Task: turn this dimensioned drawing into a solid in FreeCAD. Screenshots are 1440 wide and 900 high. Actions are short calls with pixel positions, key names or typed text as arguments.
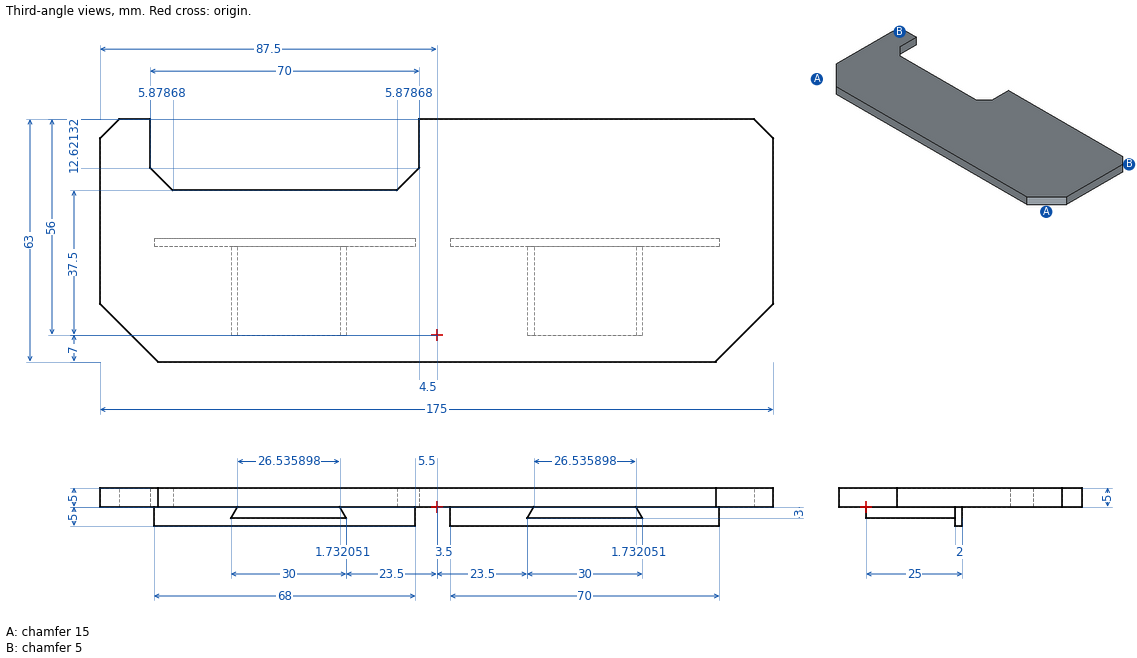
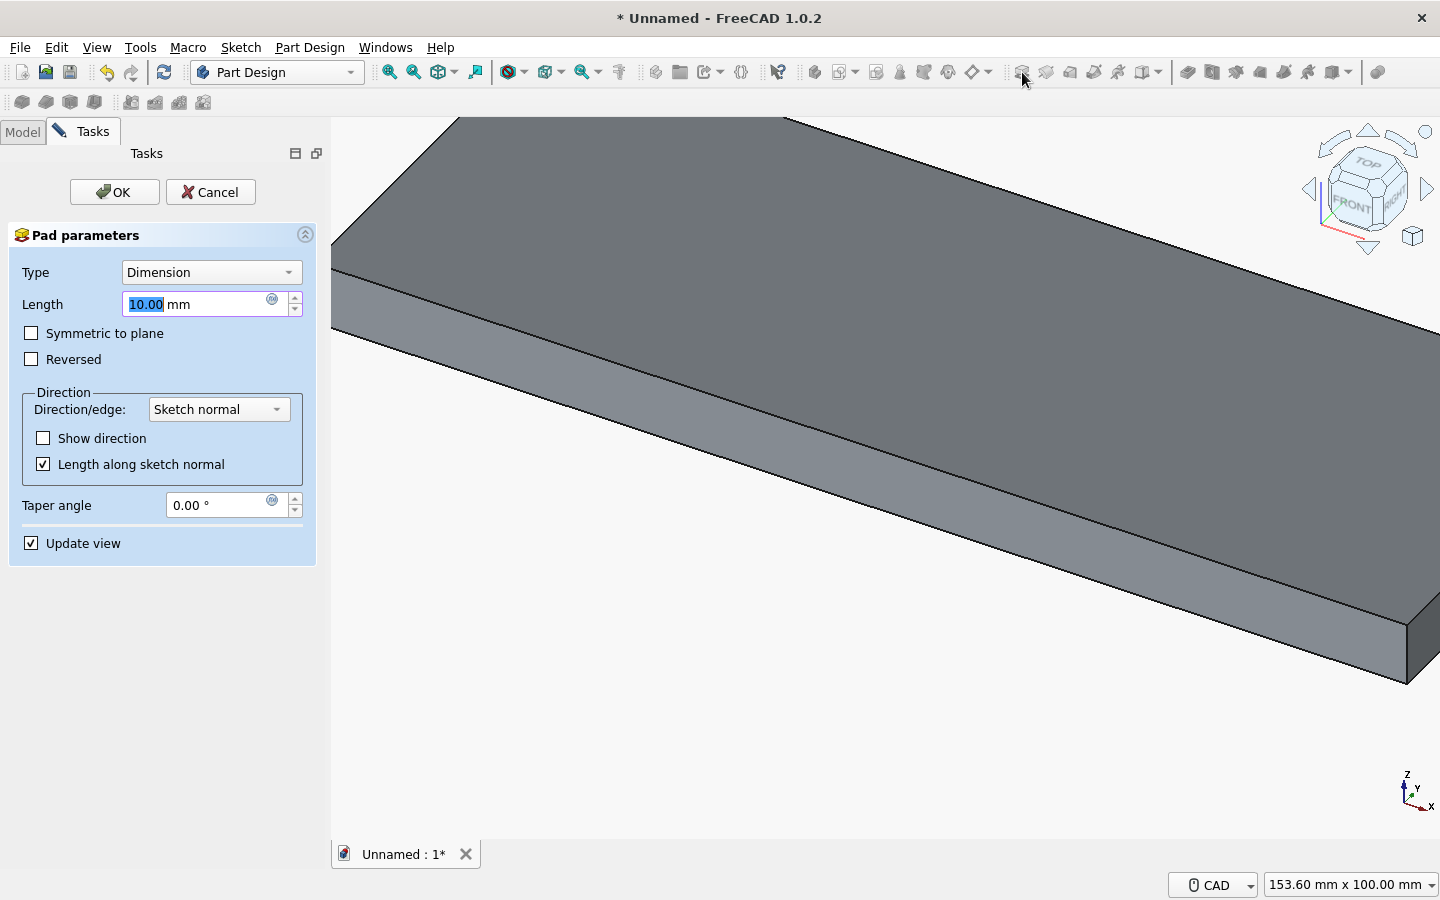
text(5)
key(Tab)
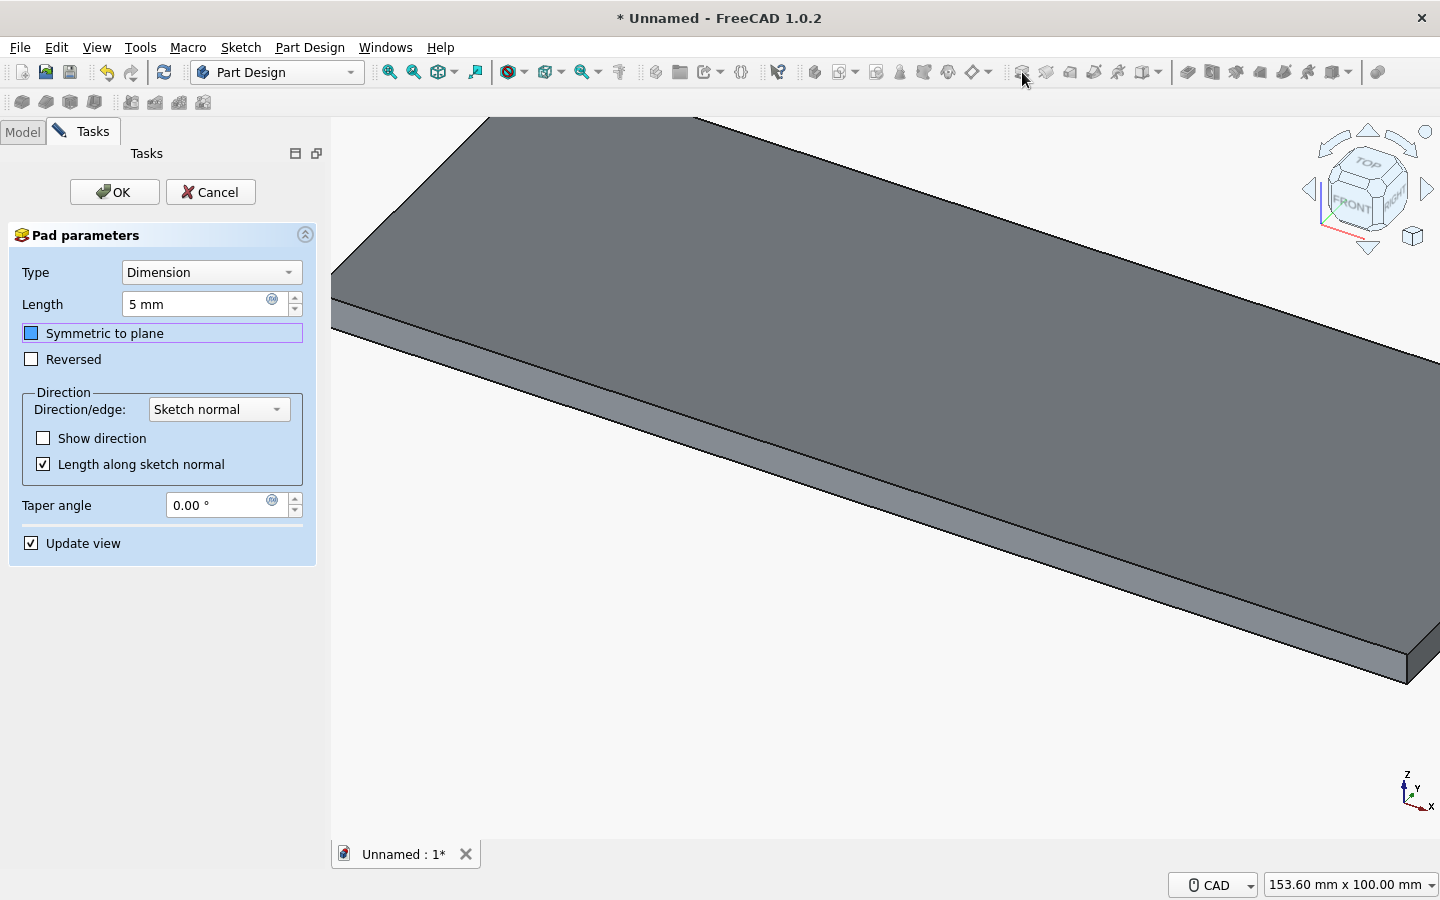
click(115, 192)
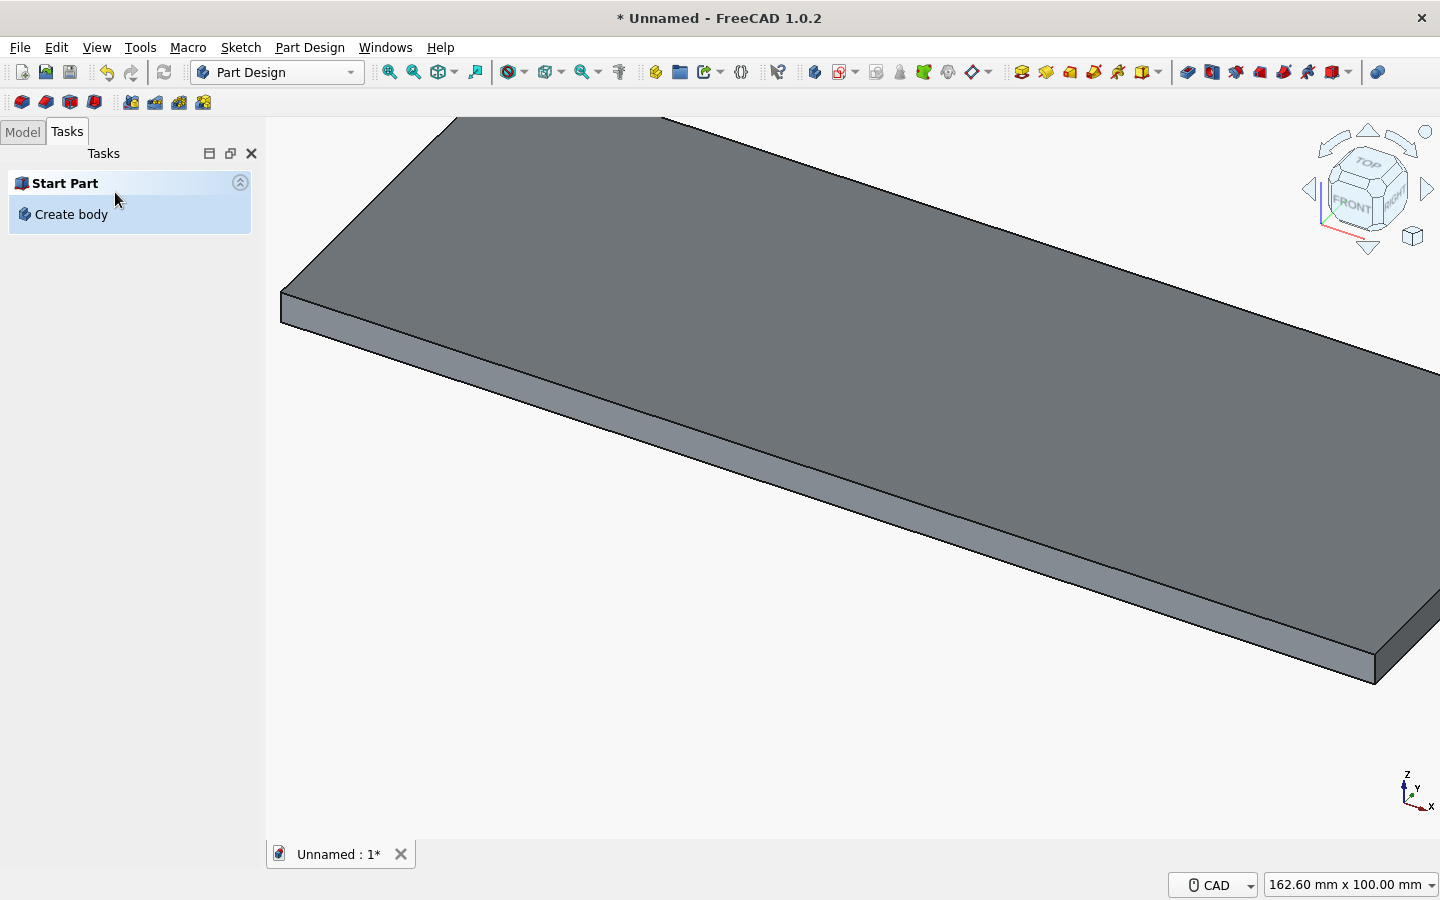
click(390, 72)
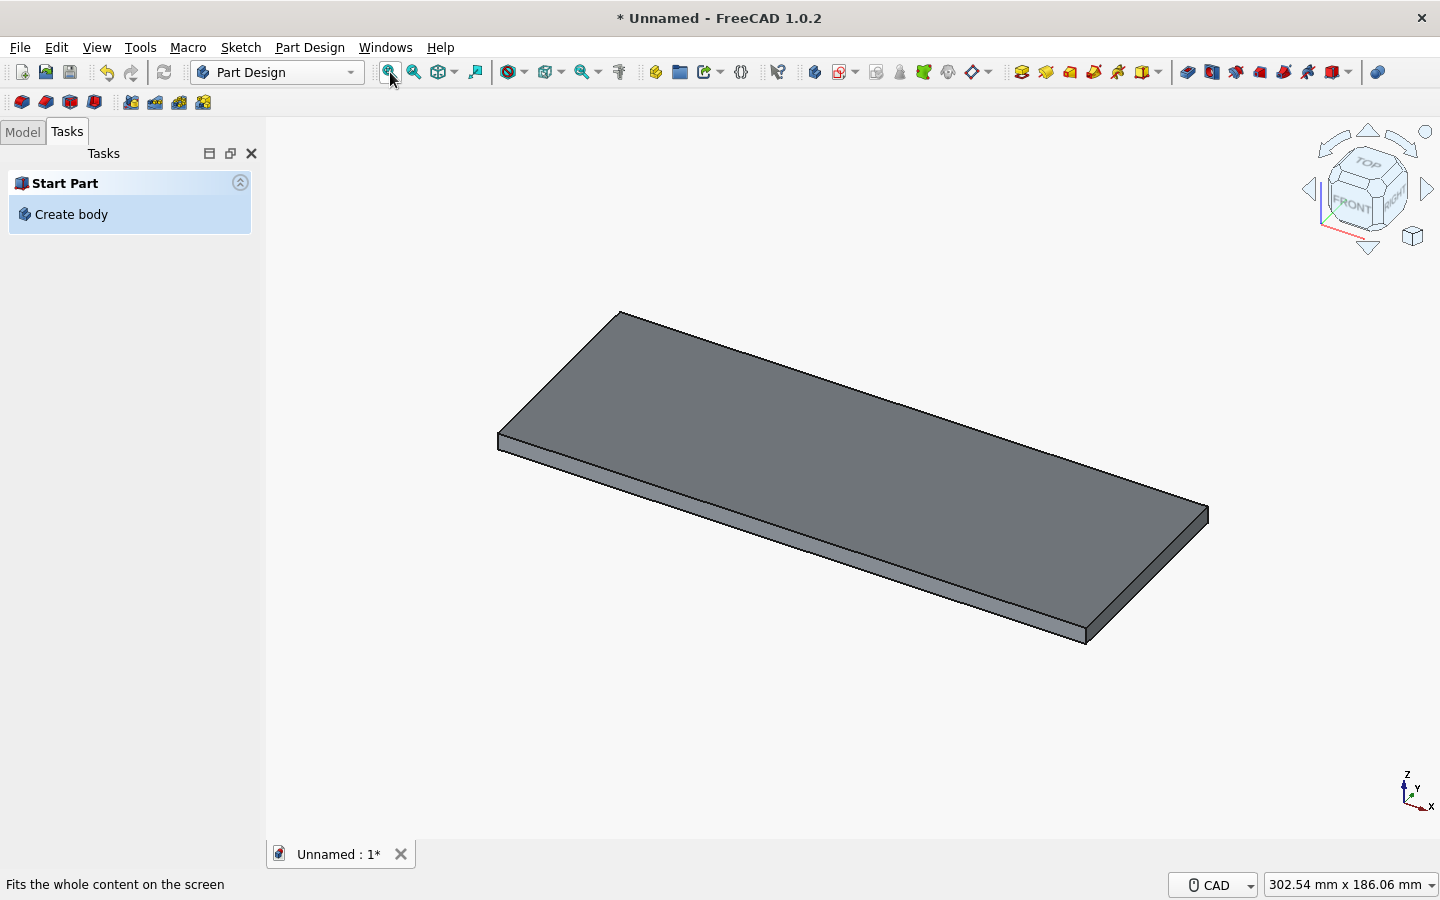
click(1021, 525)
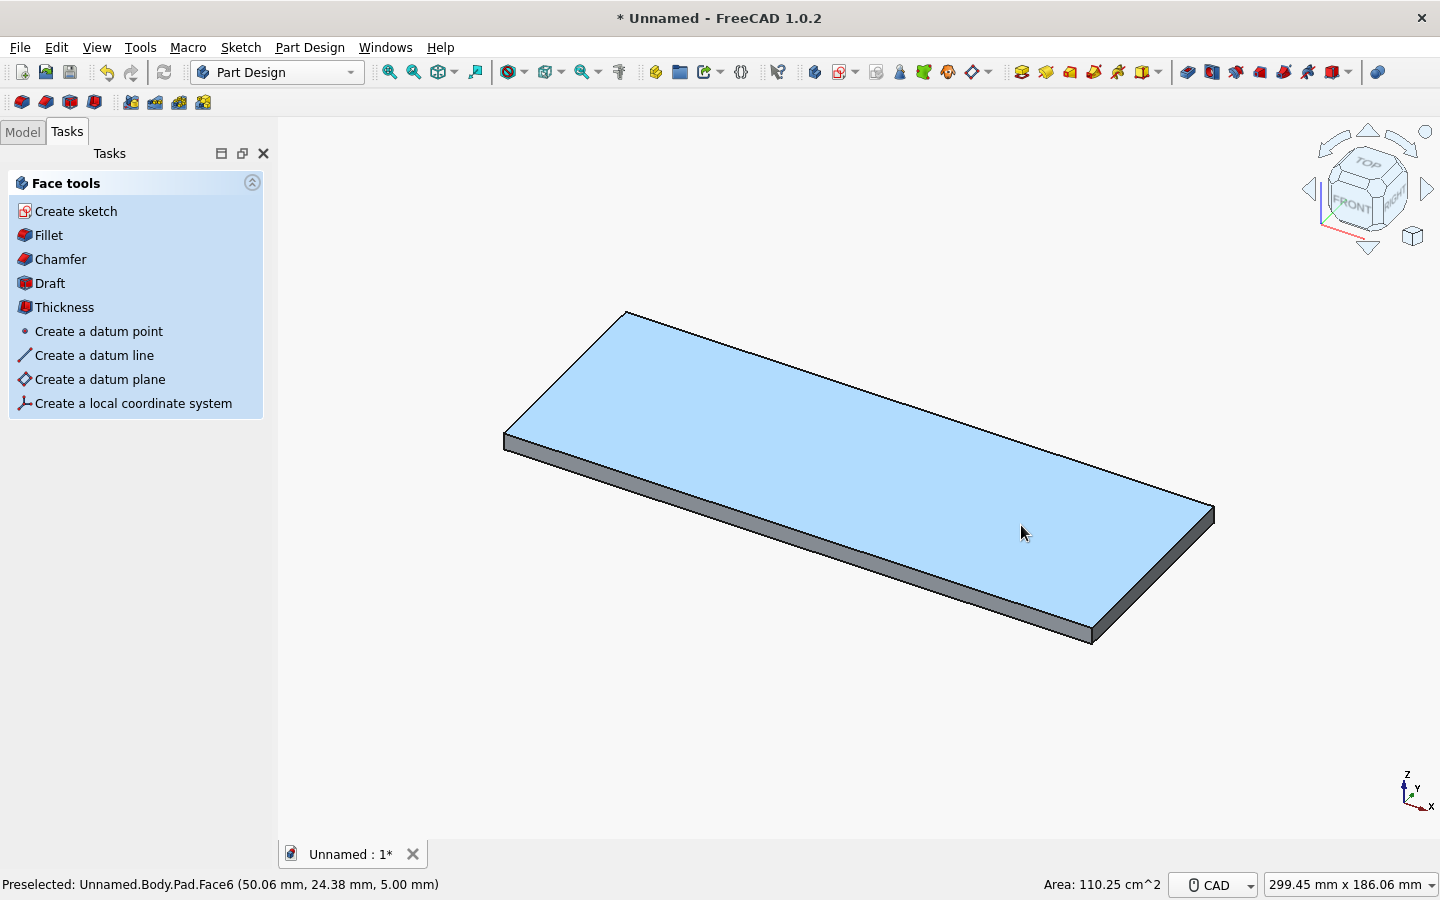
click(840, 72)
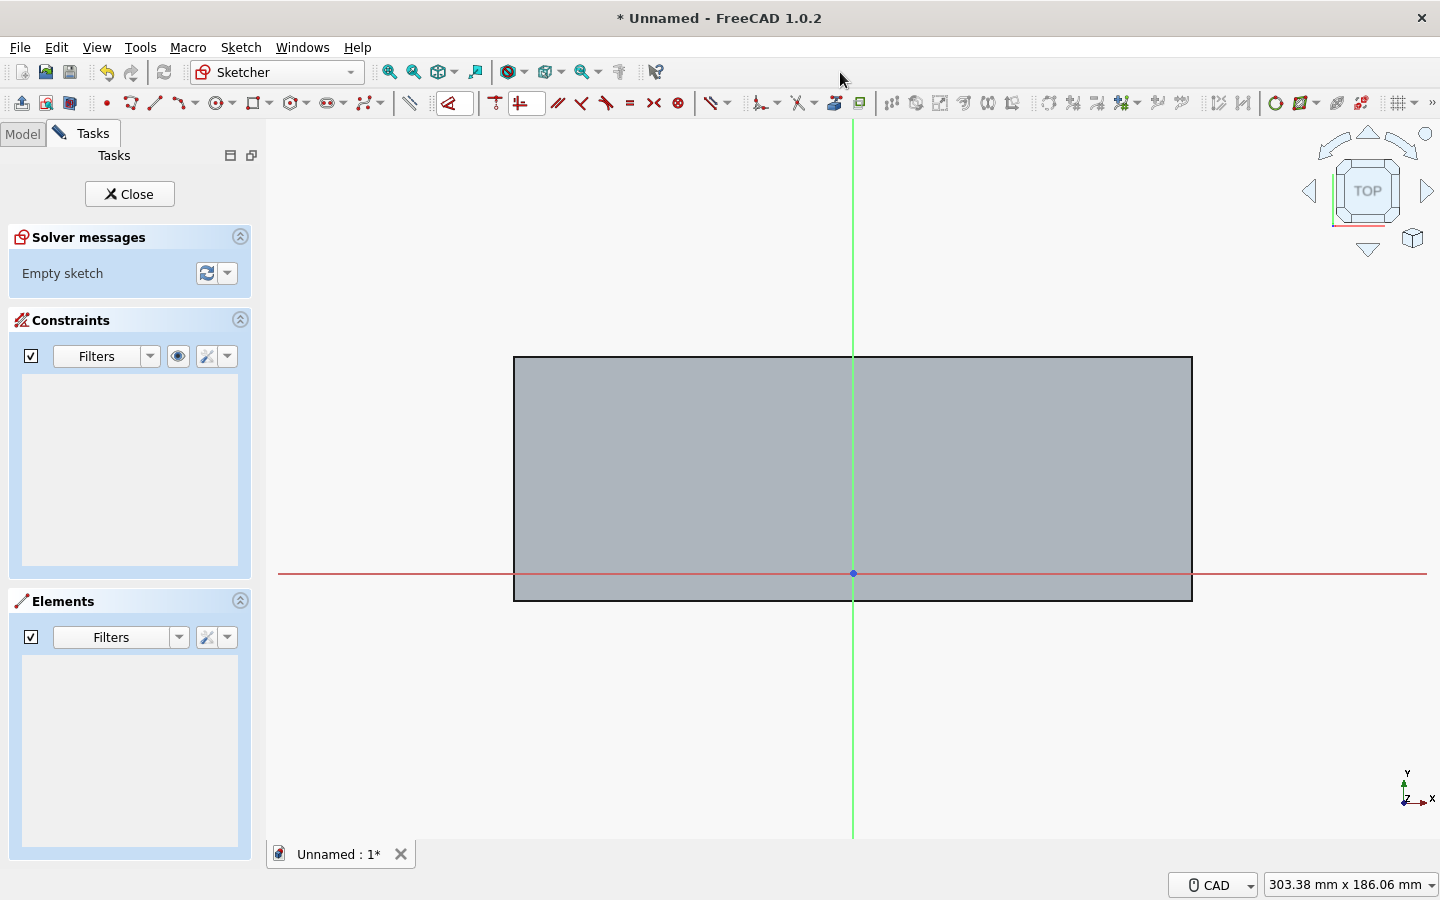
scroll(647, 454, up, 4)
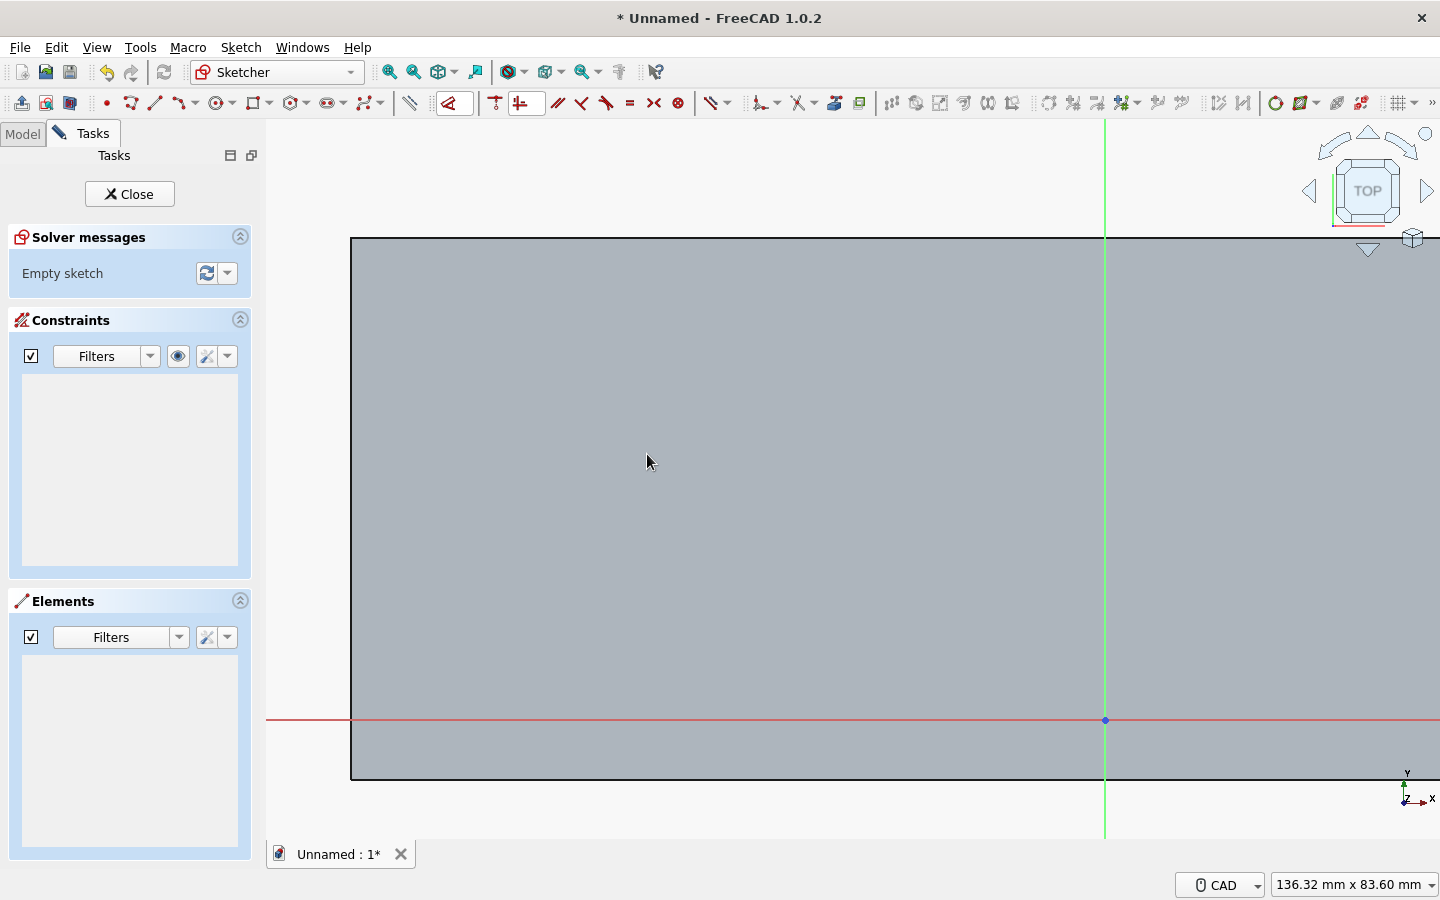
key(g)
key(m)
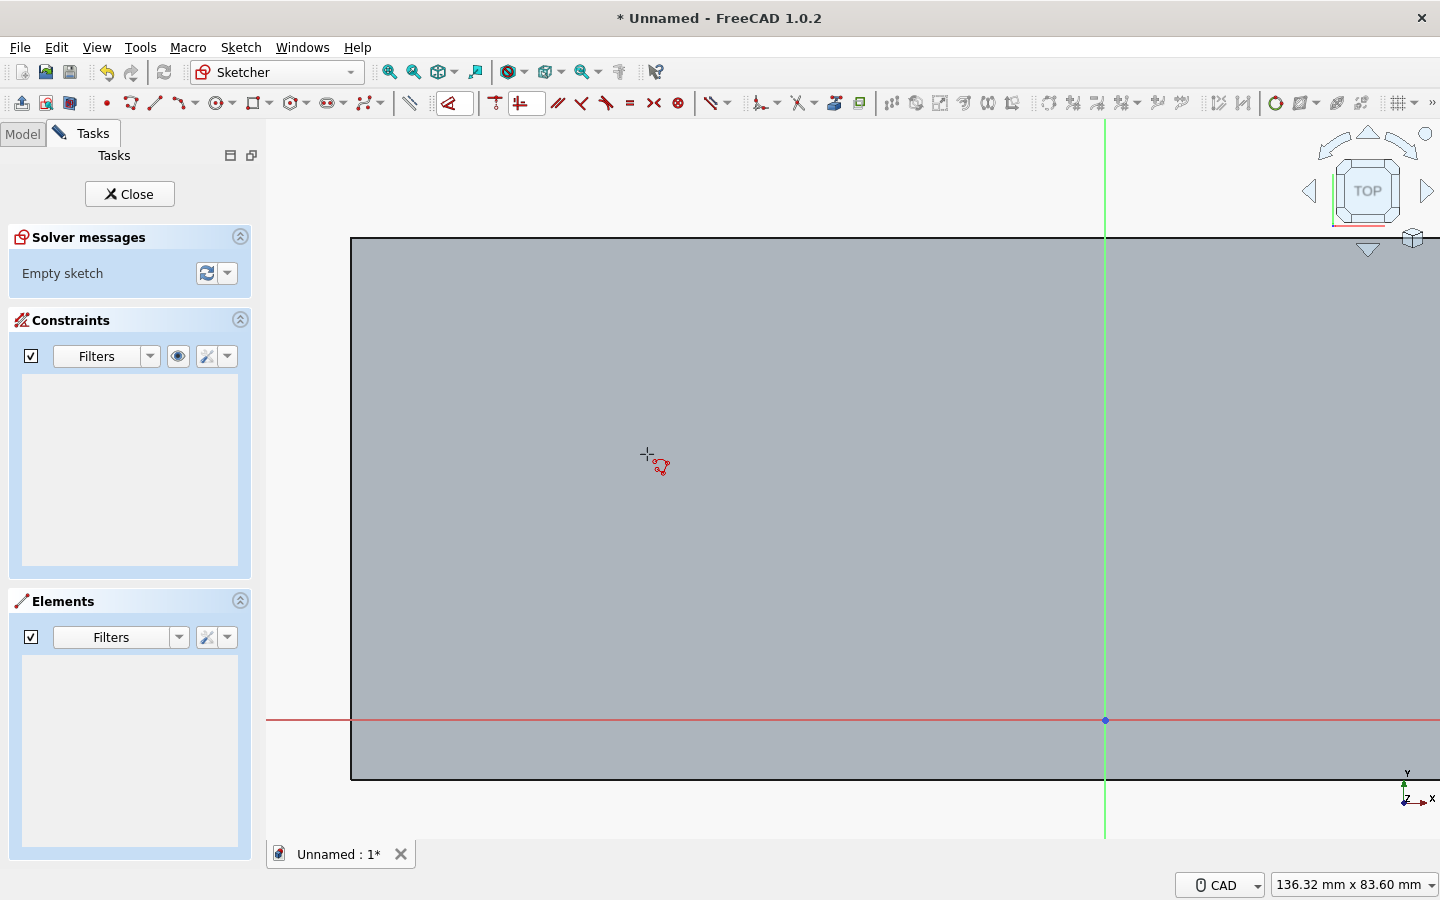
click(1016, 397)
click(1066, 346)
click(1066, 238)
click(463, 238)
click(463, 346)
click(514, 397)
click(1016, 398)
key(Escape)
key(Escape)